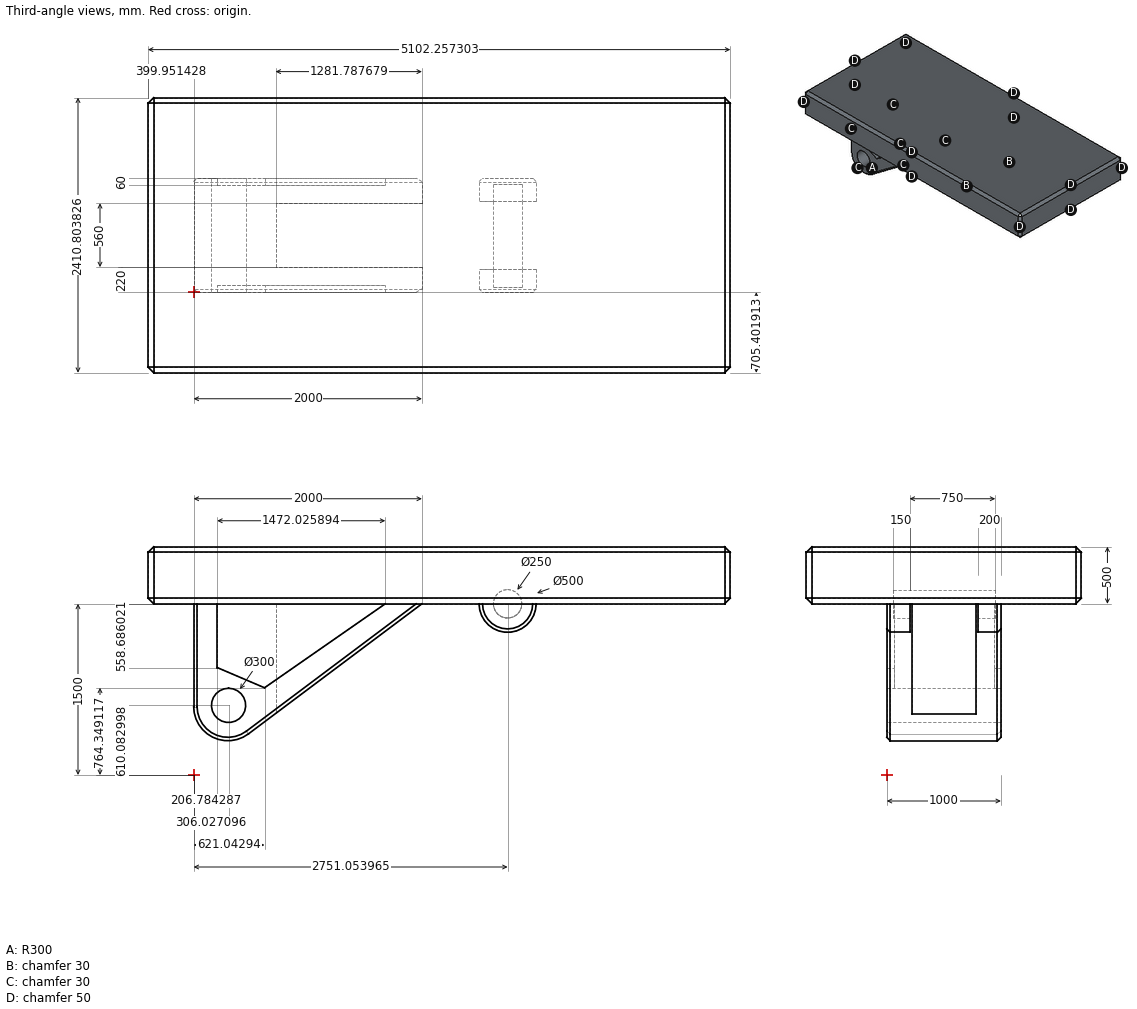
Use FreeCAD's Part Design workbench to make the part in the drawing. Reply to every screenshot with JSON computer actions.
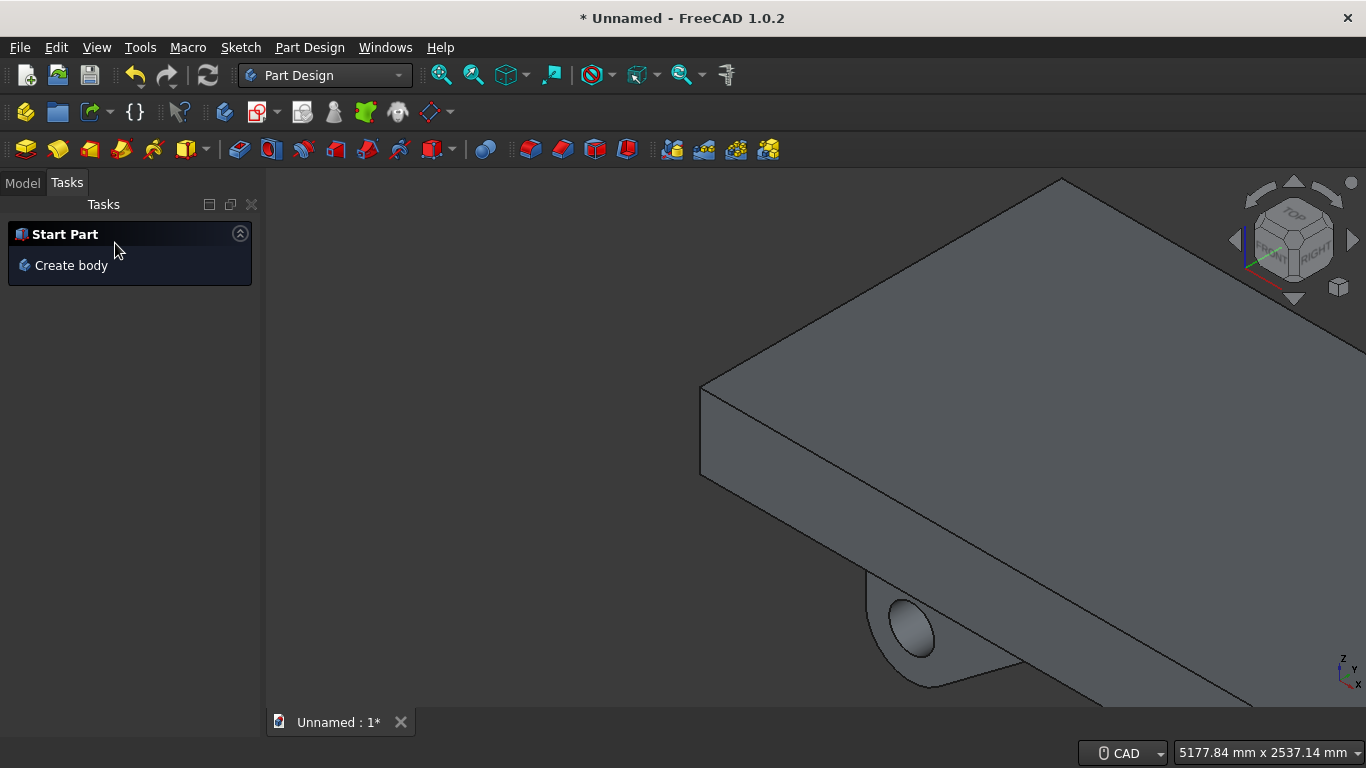
{"action": "key", "text": "v f"}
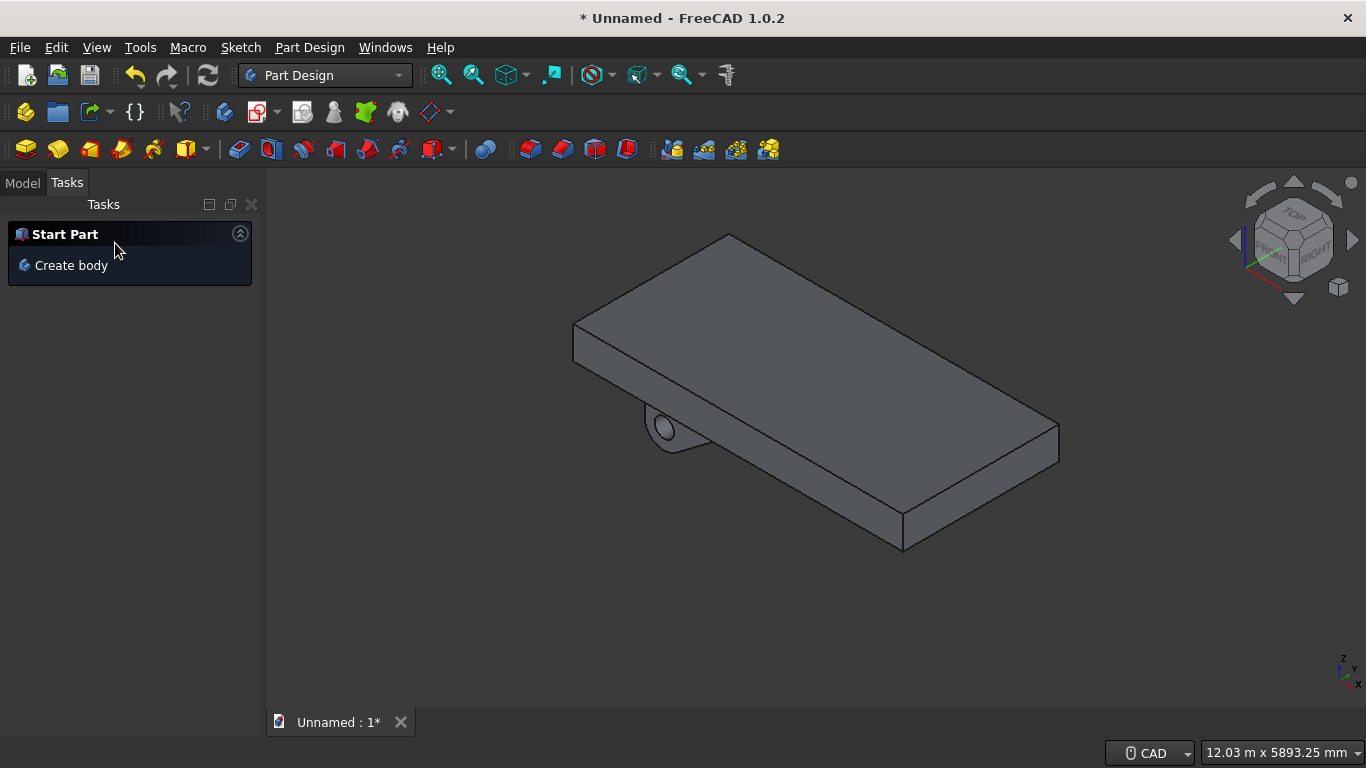
{"action": "left_click", "coordinate": [23, 182]}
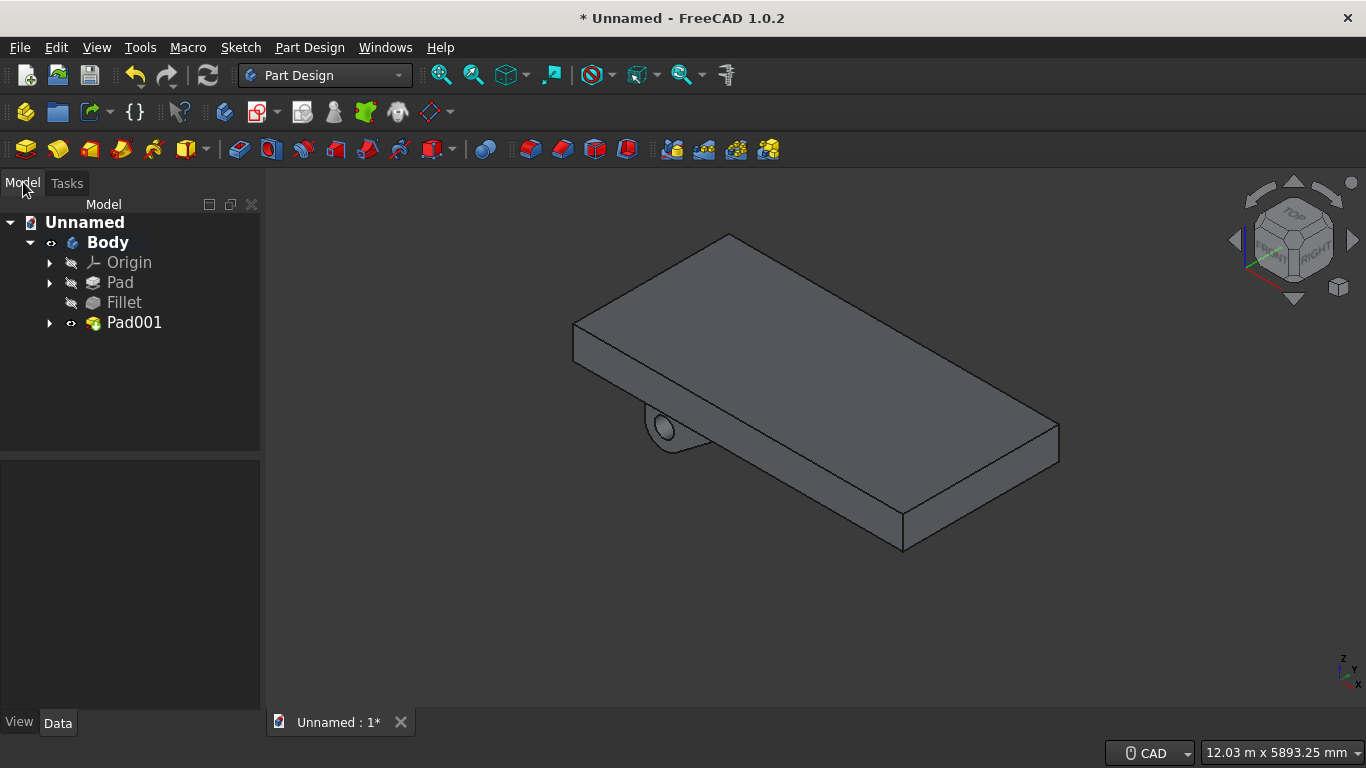
{"action": "left_click", "coordinate": [50, 263]}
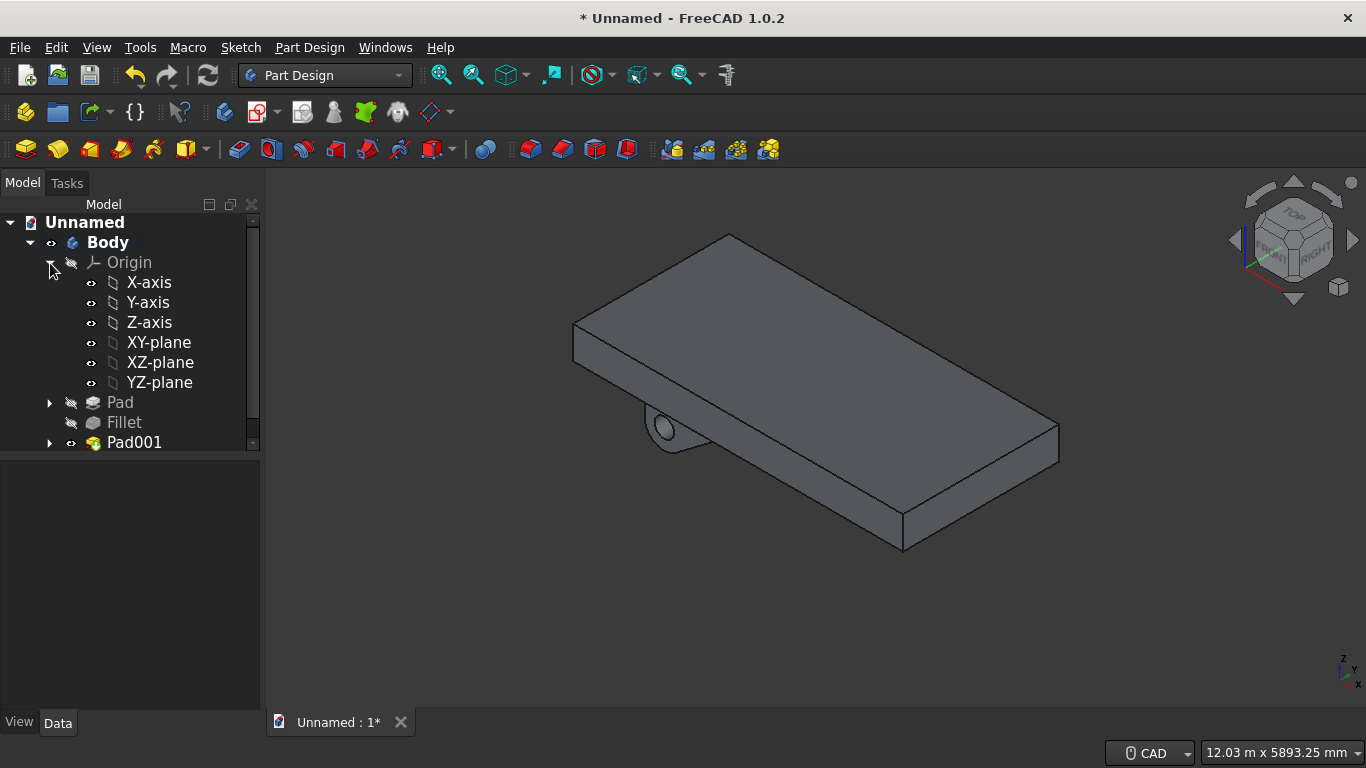
{"action": "left_click", "coordinate": [136, 363]}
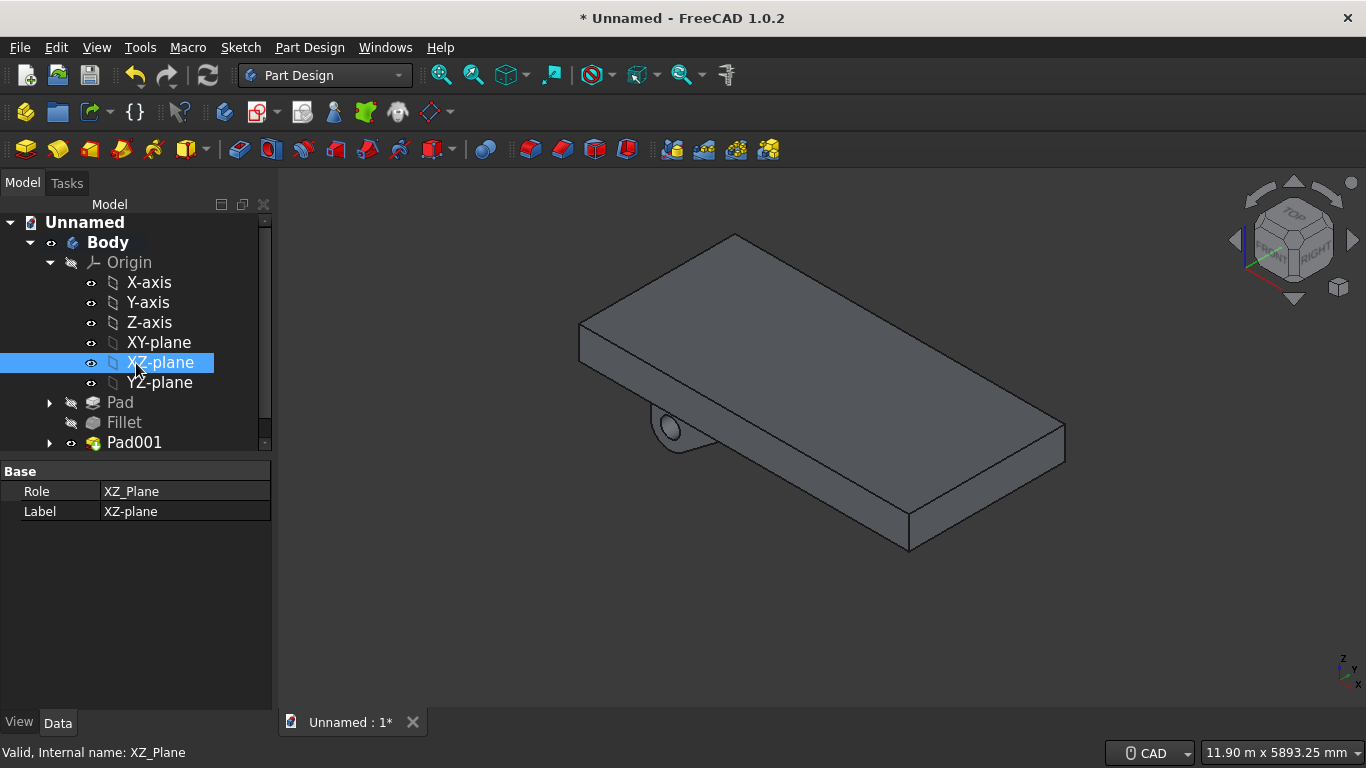
{"action": "left_click", "coordinate": [430, 112]}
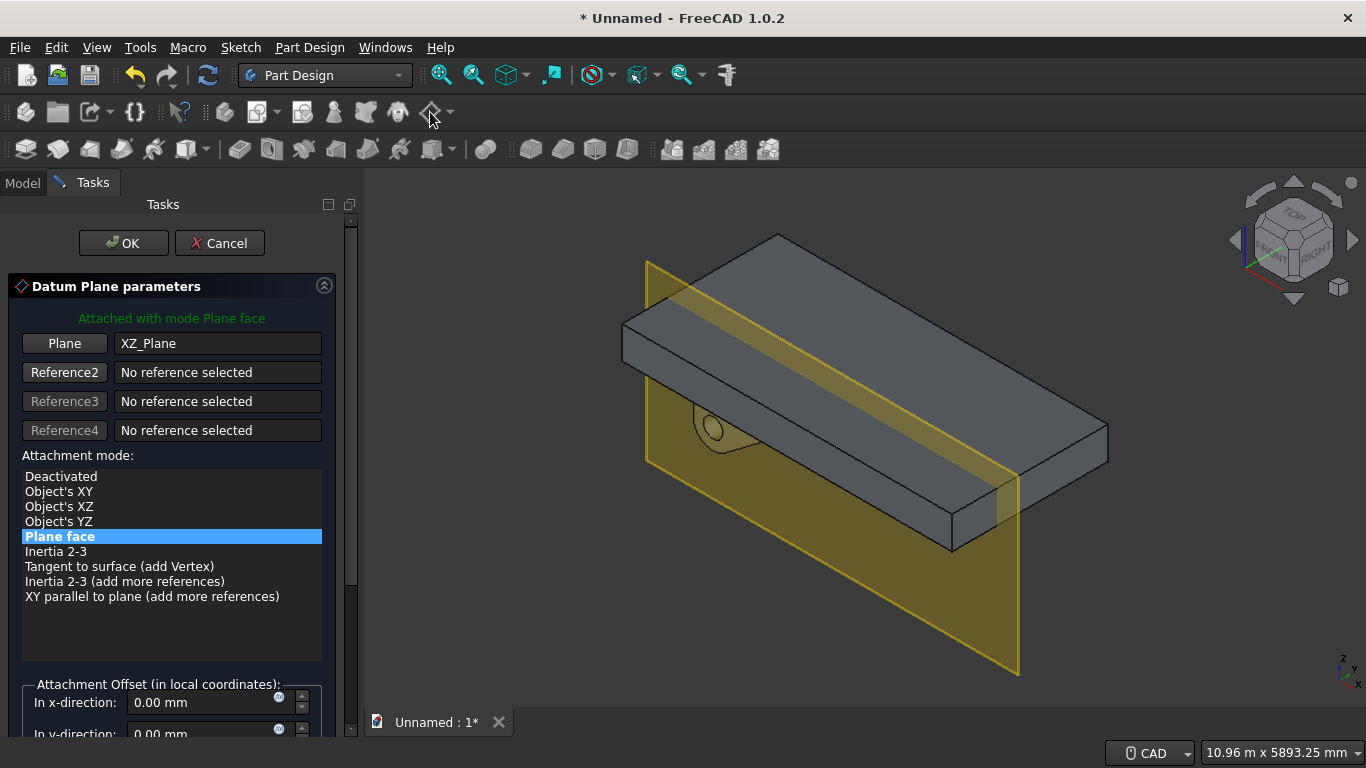
{"action": "scroll", "coordinate": [351, 475], "scroll_direction": "down", "scroll_amount": 2}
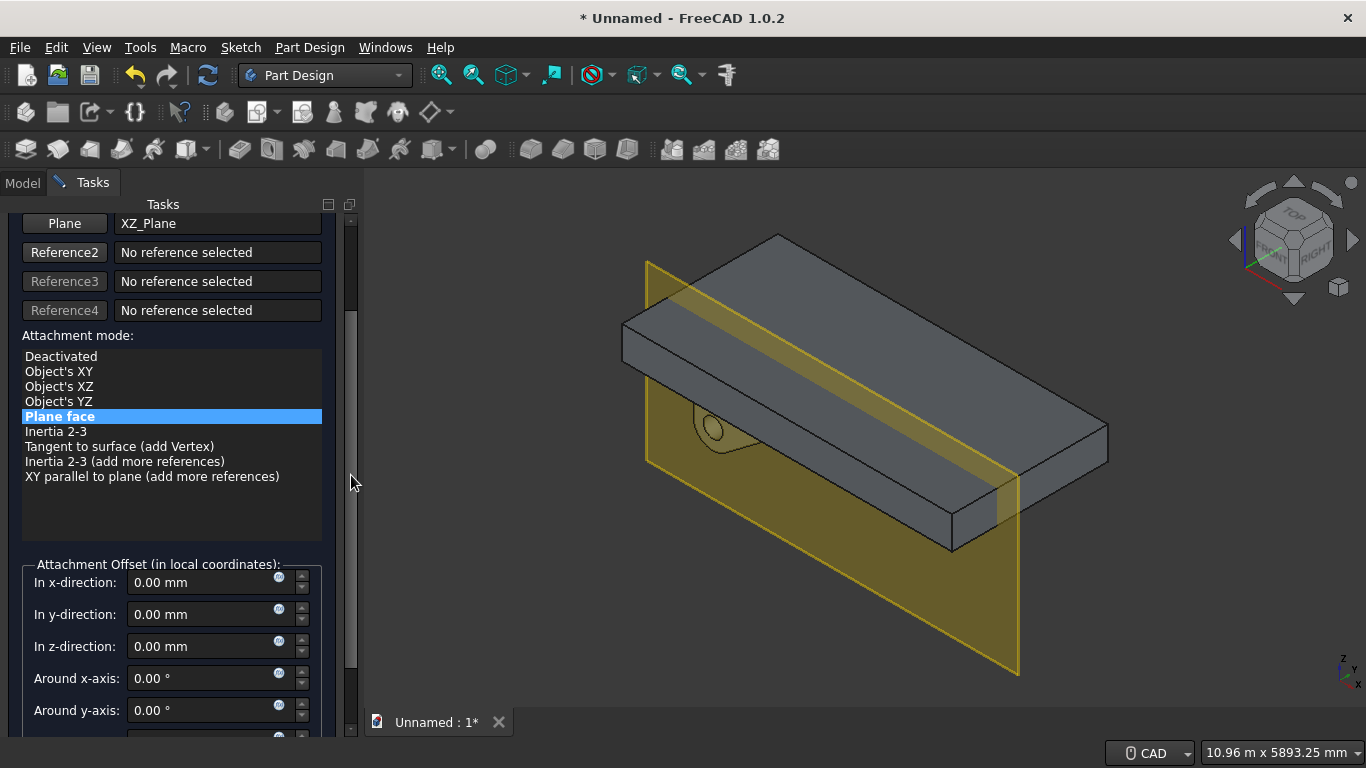
{"action": "triple_click", "coordinate": [210, 646]}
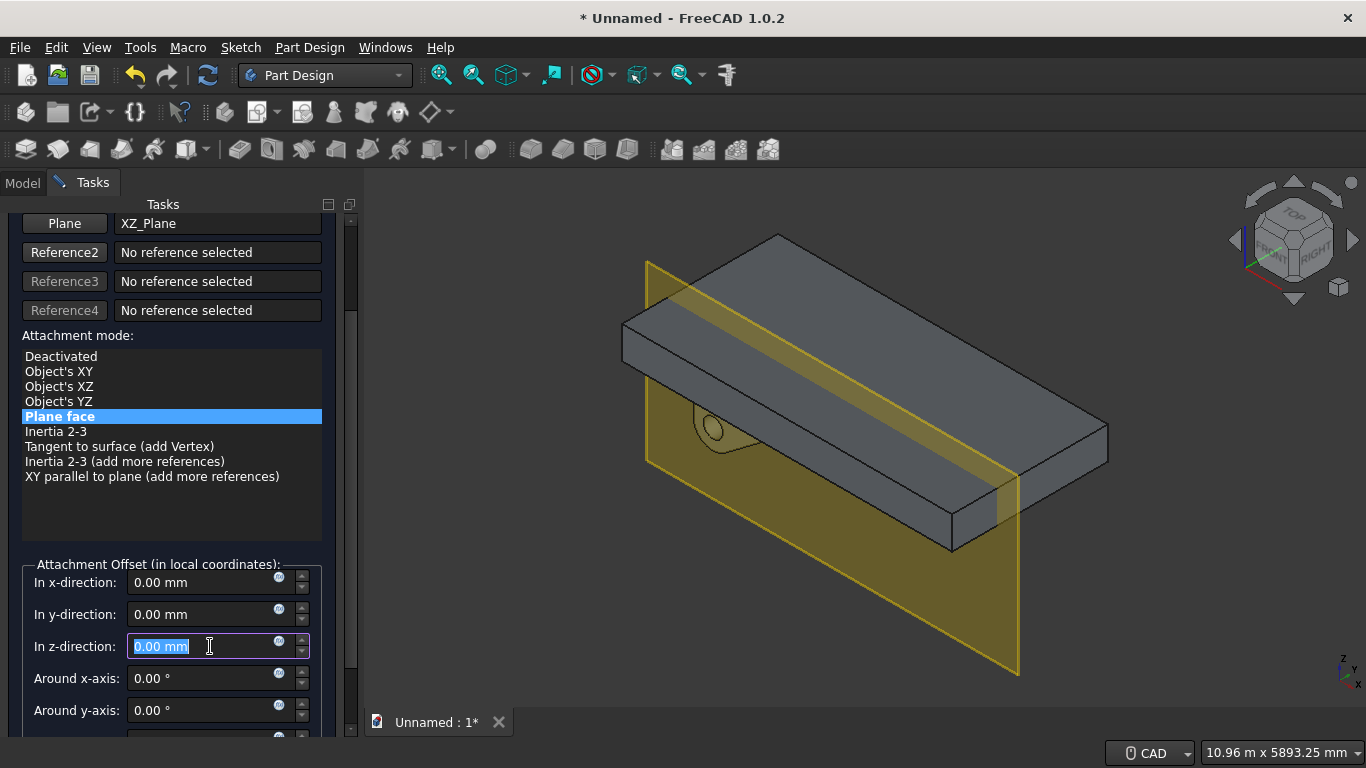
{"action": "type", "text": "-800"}
{"action": "key", "text": "Tab"}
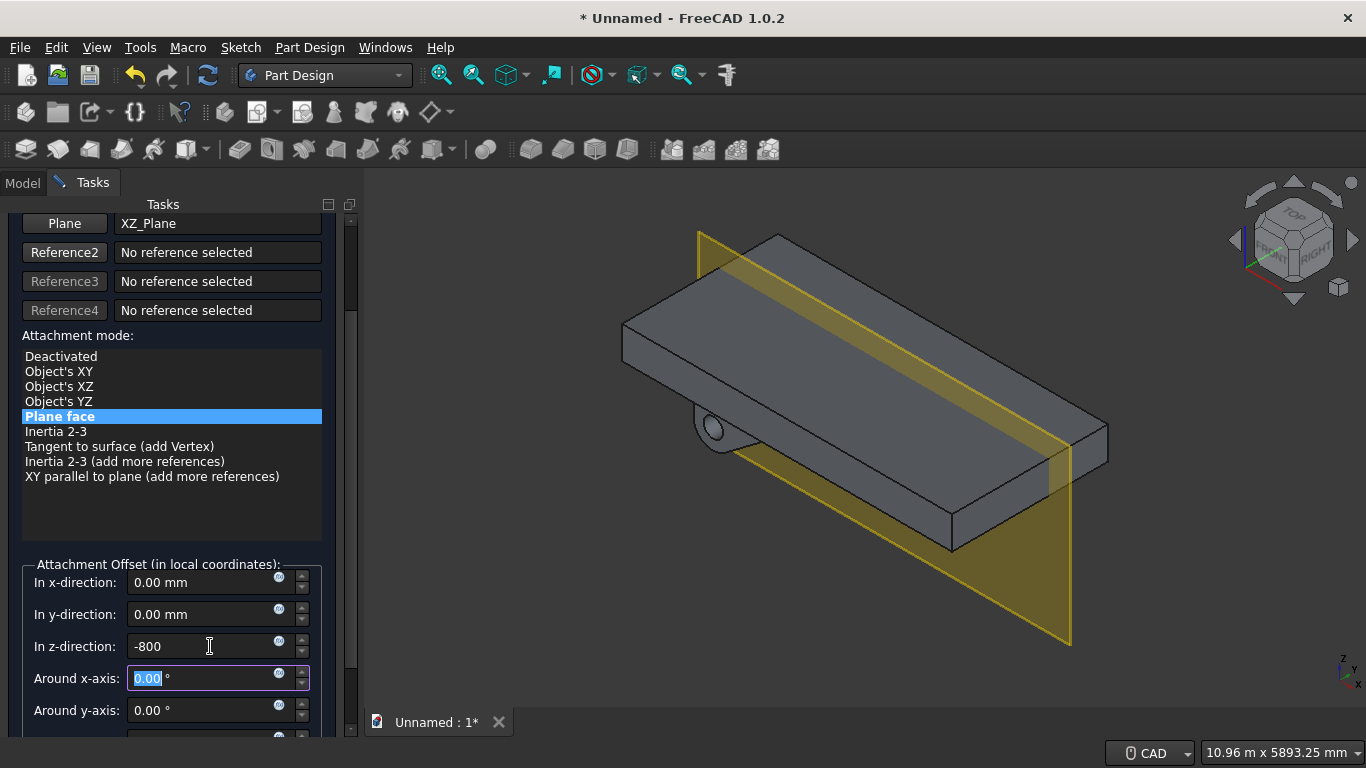
{"action": "scroll", "coordinate": [351, 475], "scroll_direction": "up", "scroll_amount": 3}